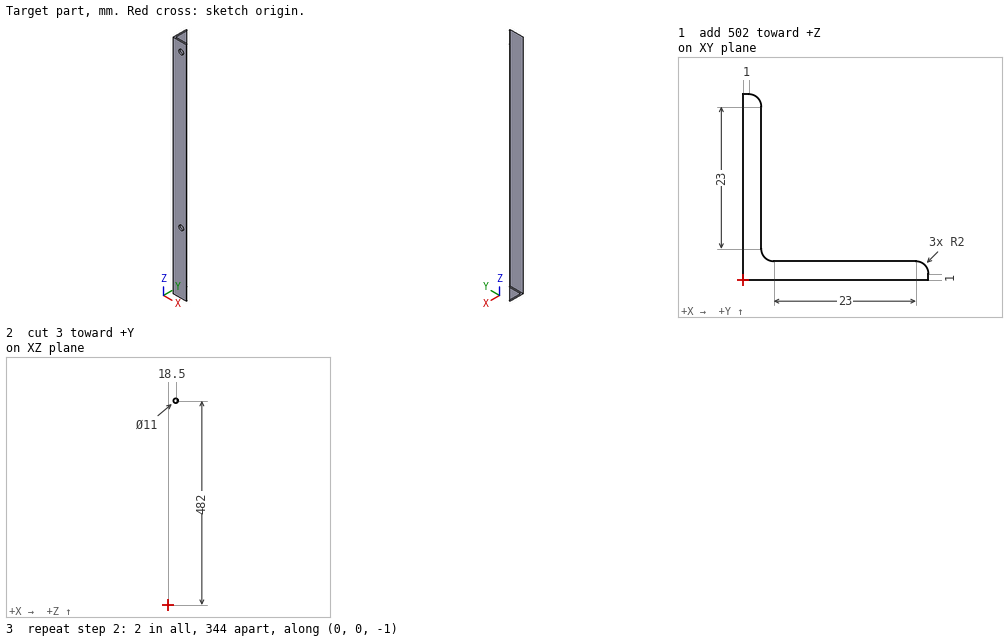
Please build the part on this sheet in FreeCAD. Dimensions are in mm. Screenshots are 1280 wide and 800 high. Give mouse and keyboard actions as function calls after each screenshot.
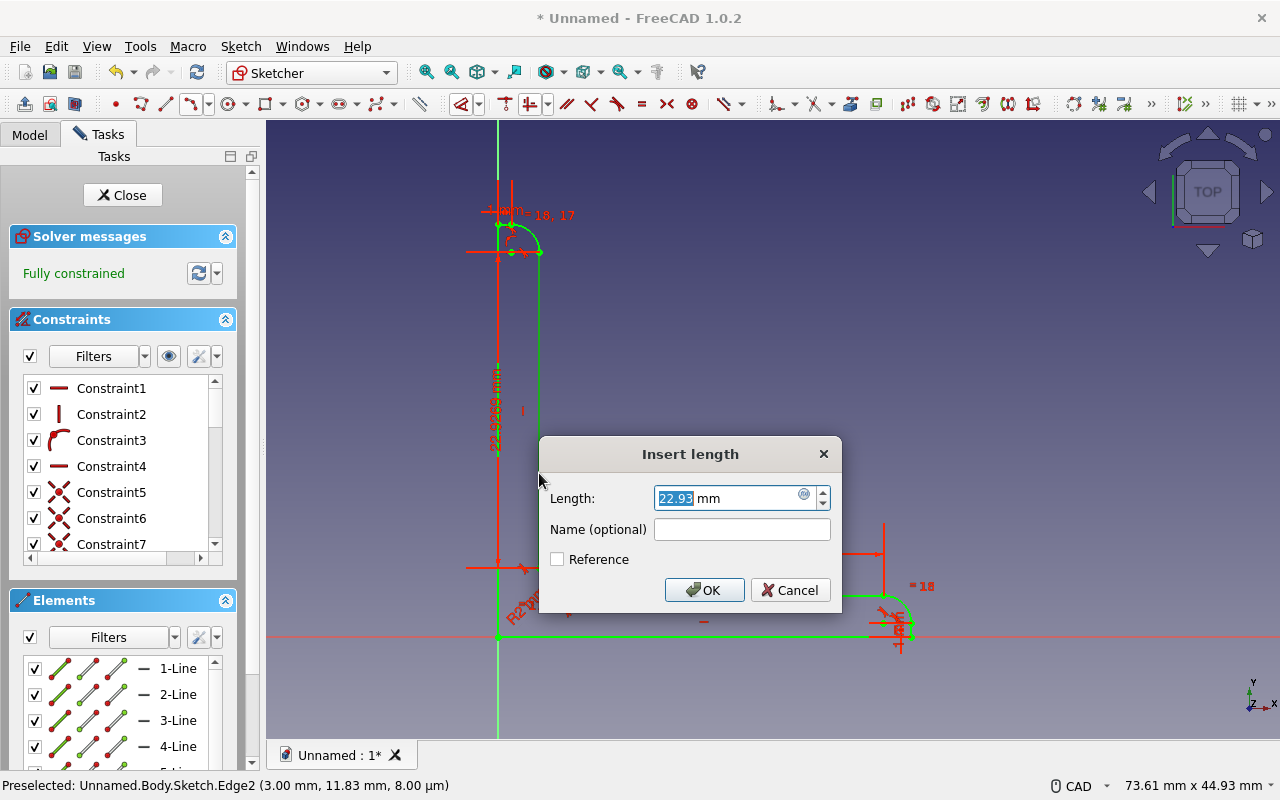
text(23)
key(Return)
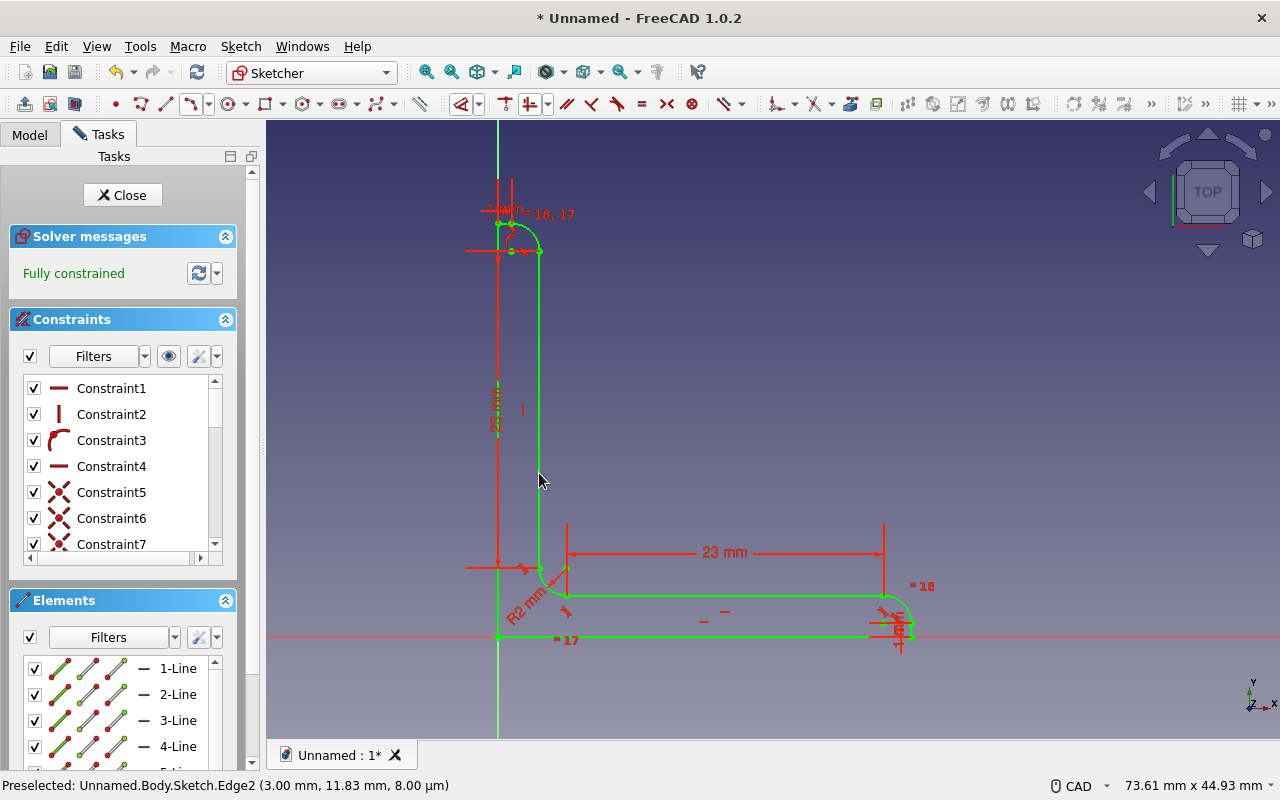
click(123, 195)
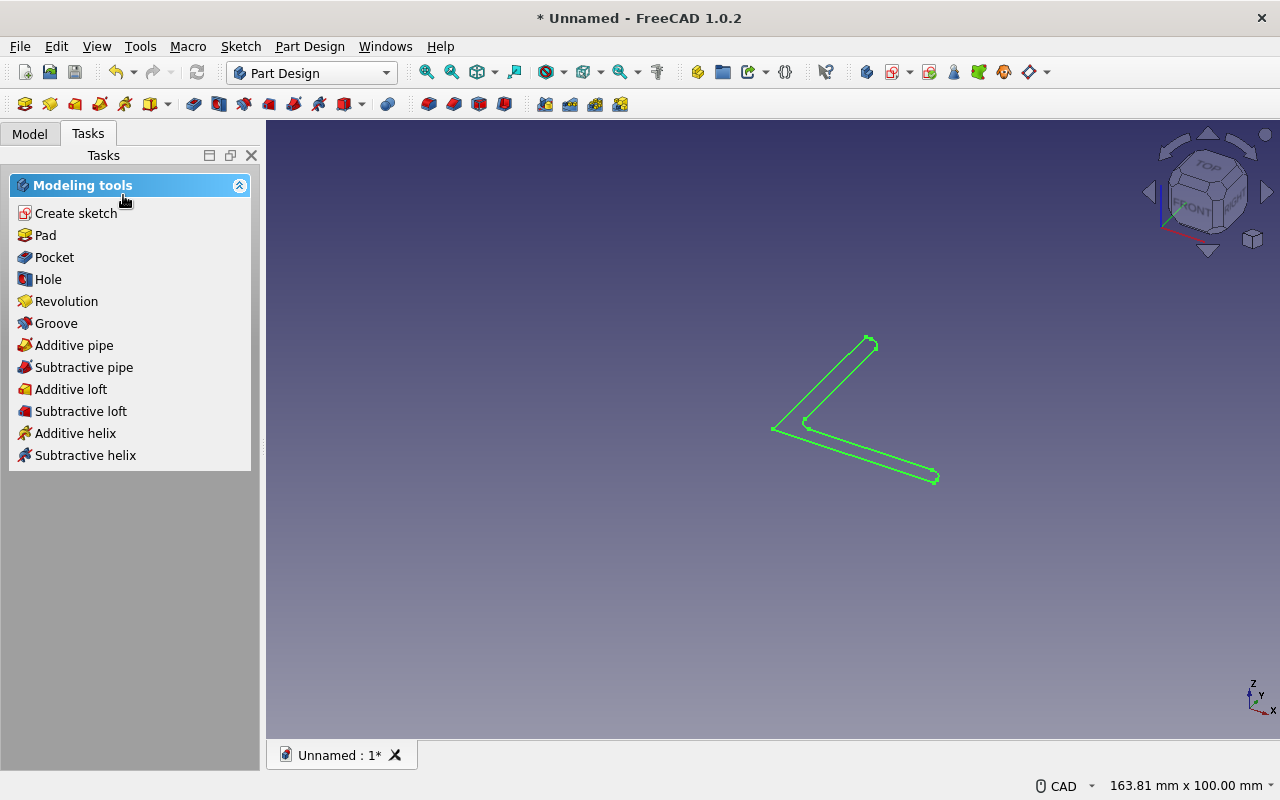
click(25, 104)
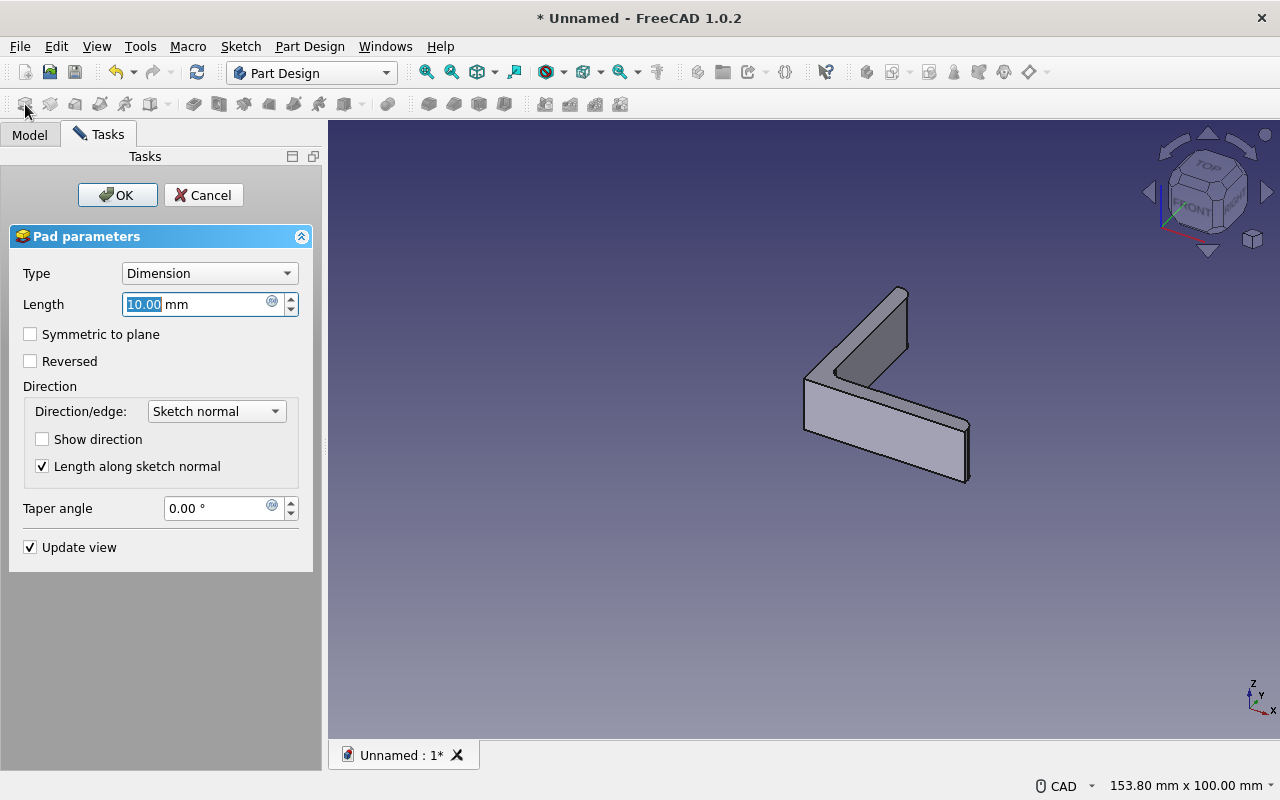
text(502)
key(Tab)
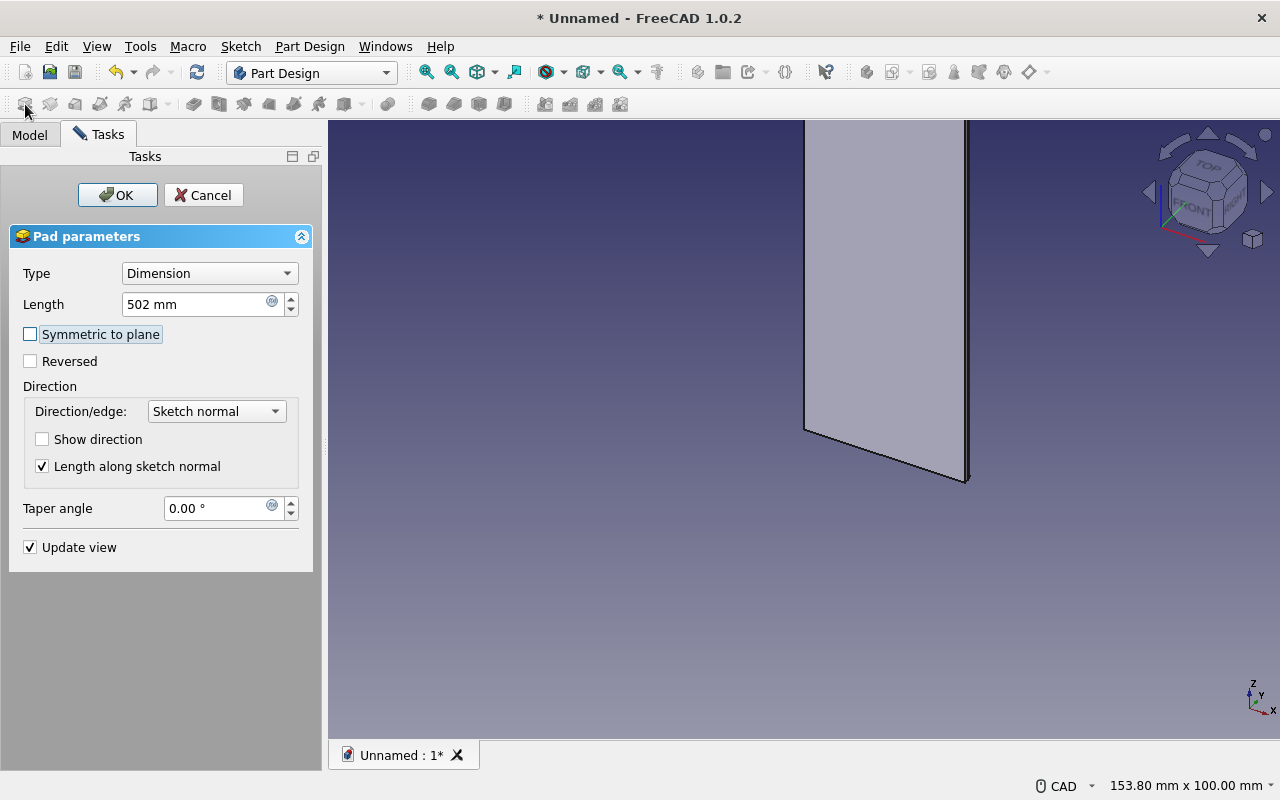
click(118, 195)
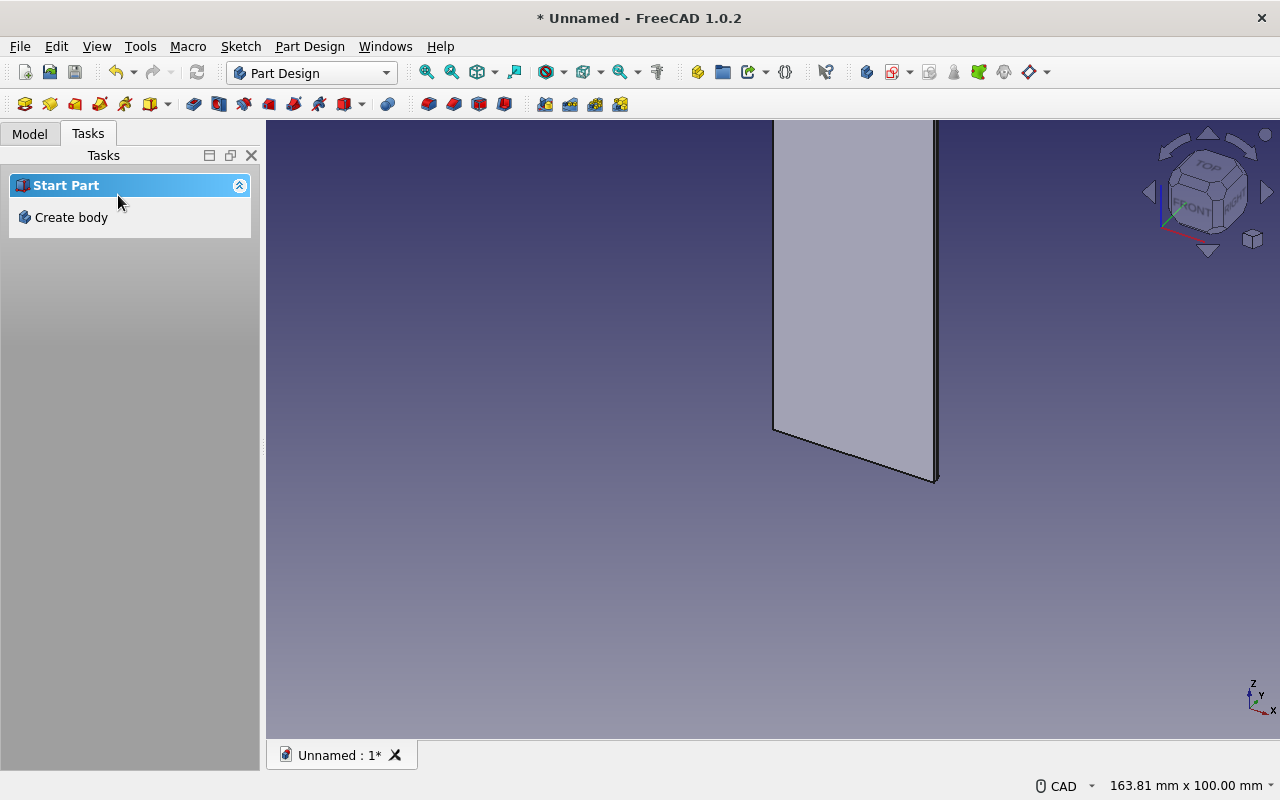
key(v)
key(f)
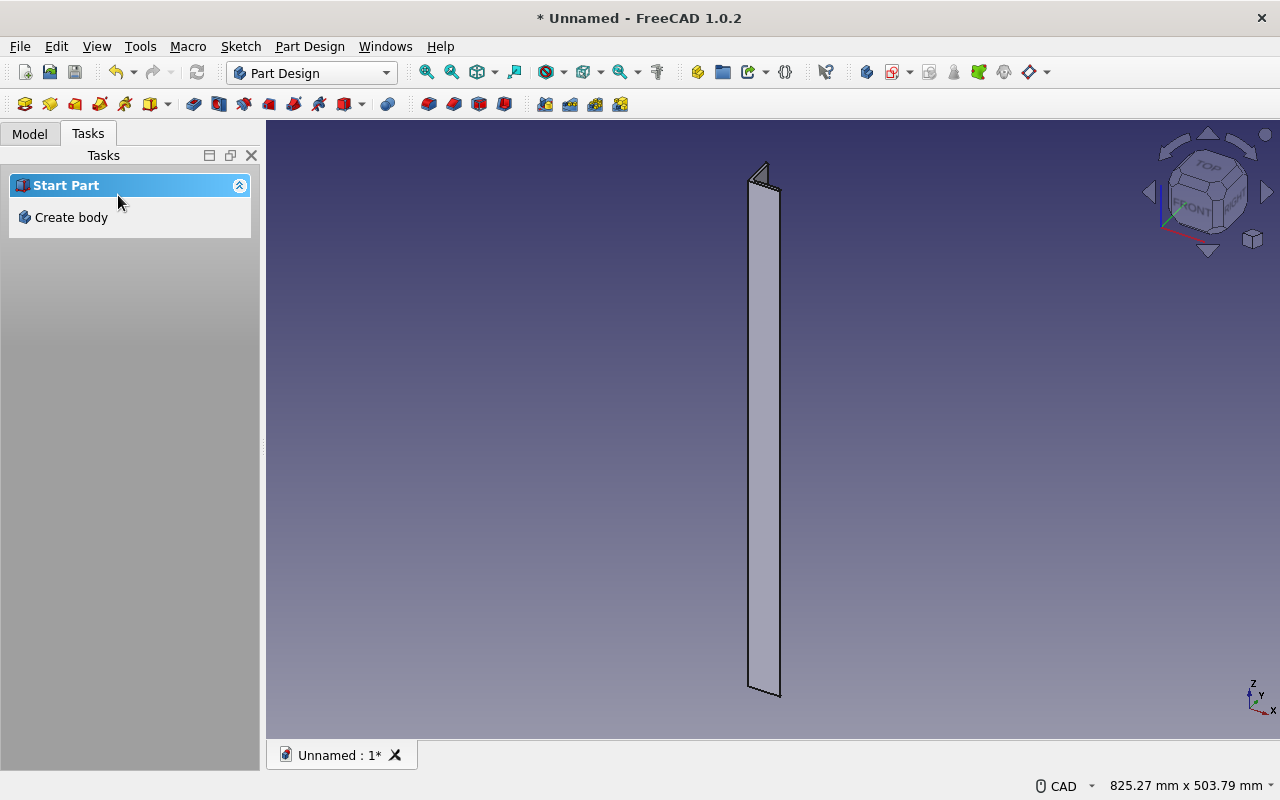
click(892, 72)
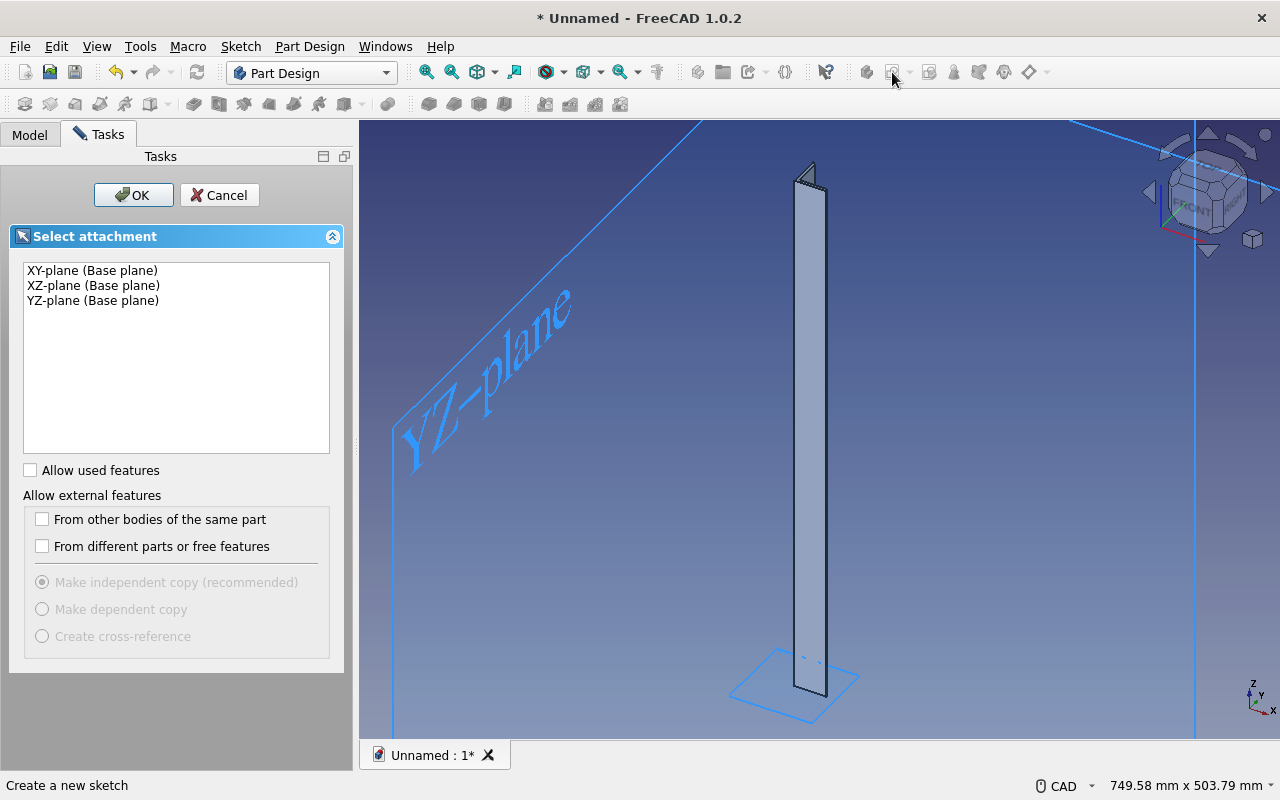
click(84, 286)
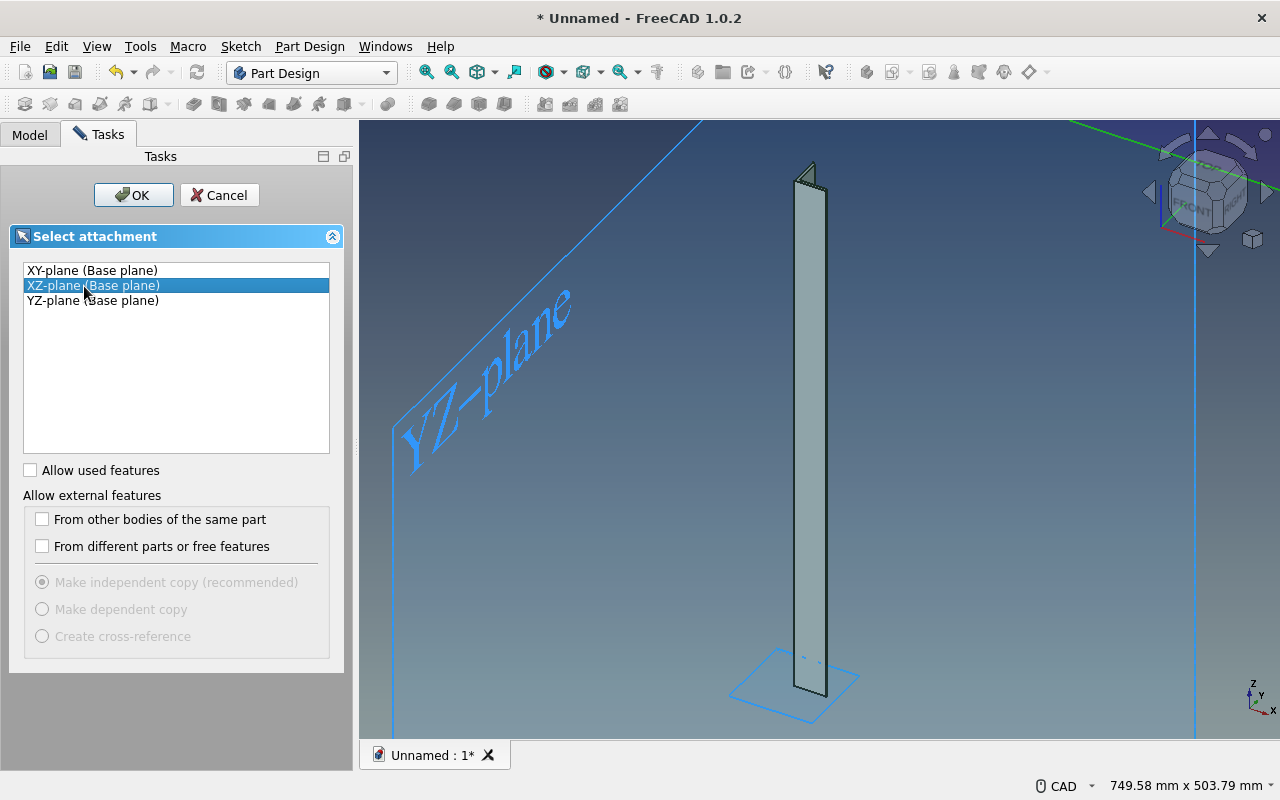
click(134, 195)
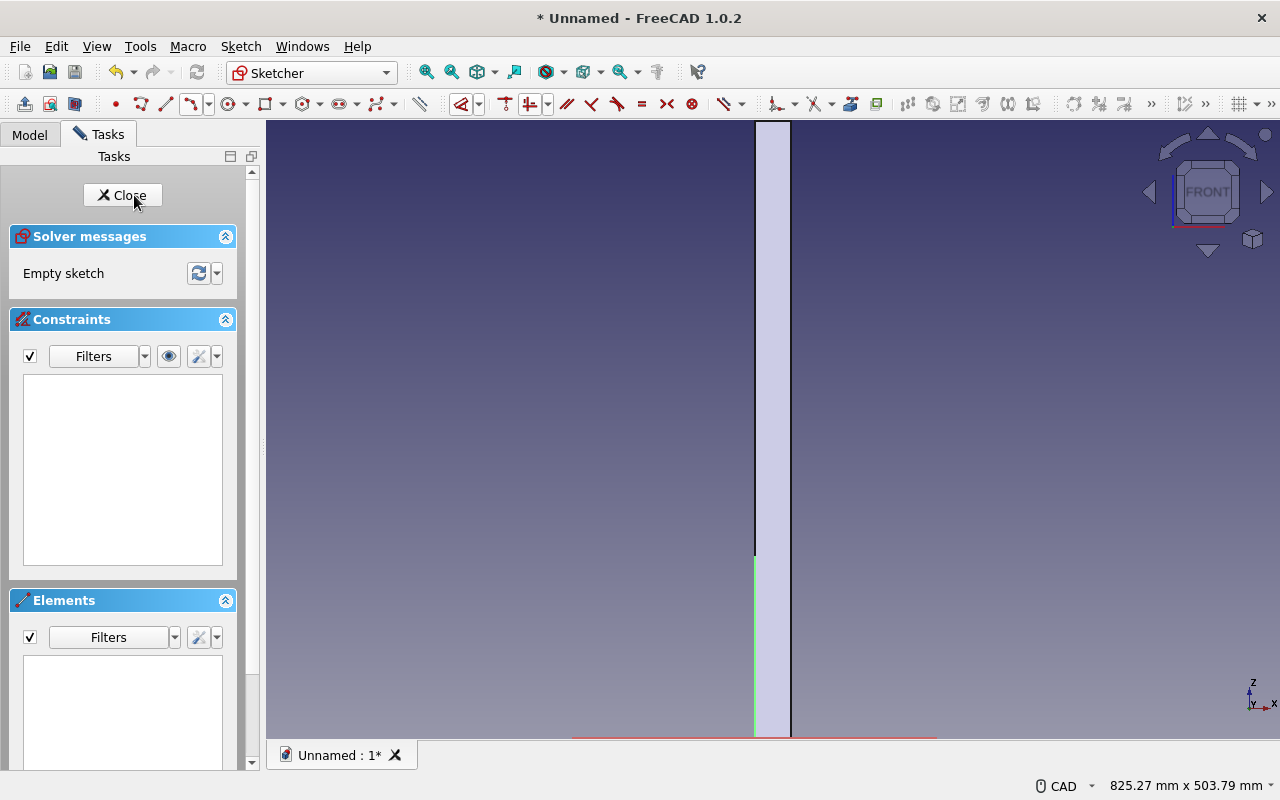
scroll(704, 430, down, 5)